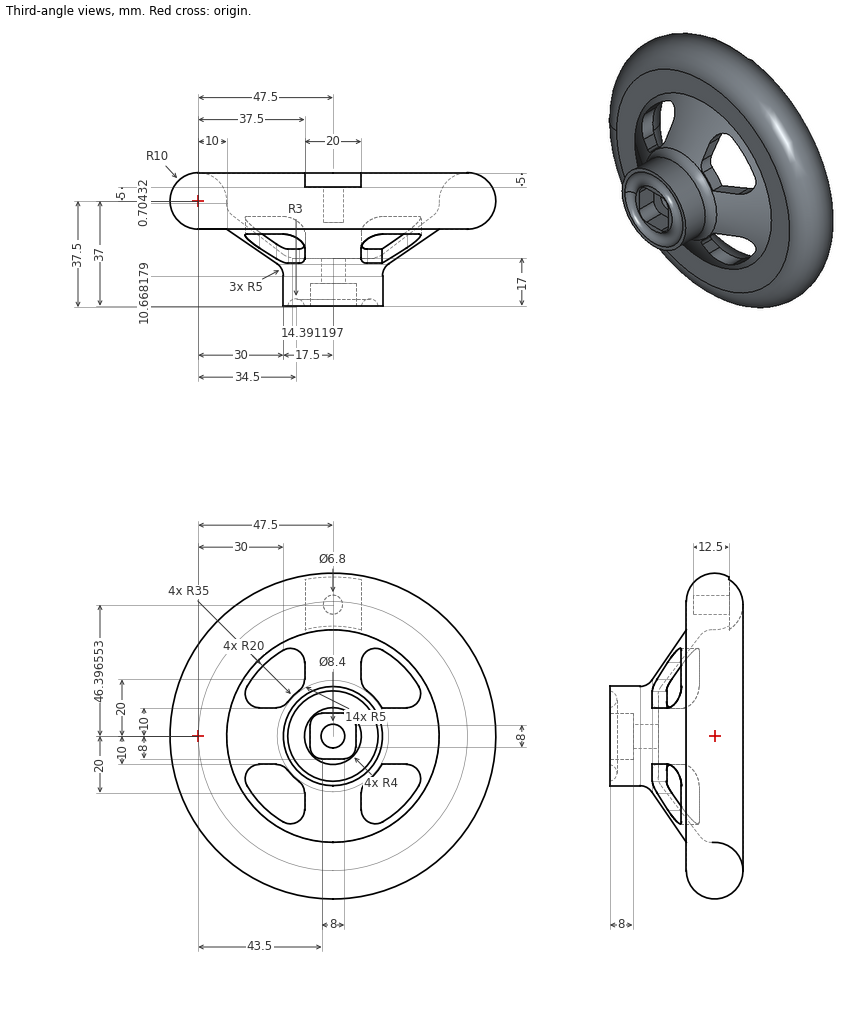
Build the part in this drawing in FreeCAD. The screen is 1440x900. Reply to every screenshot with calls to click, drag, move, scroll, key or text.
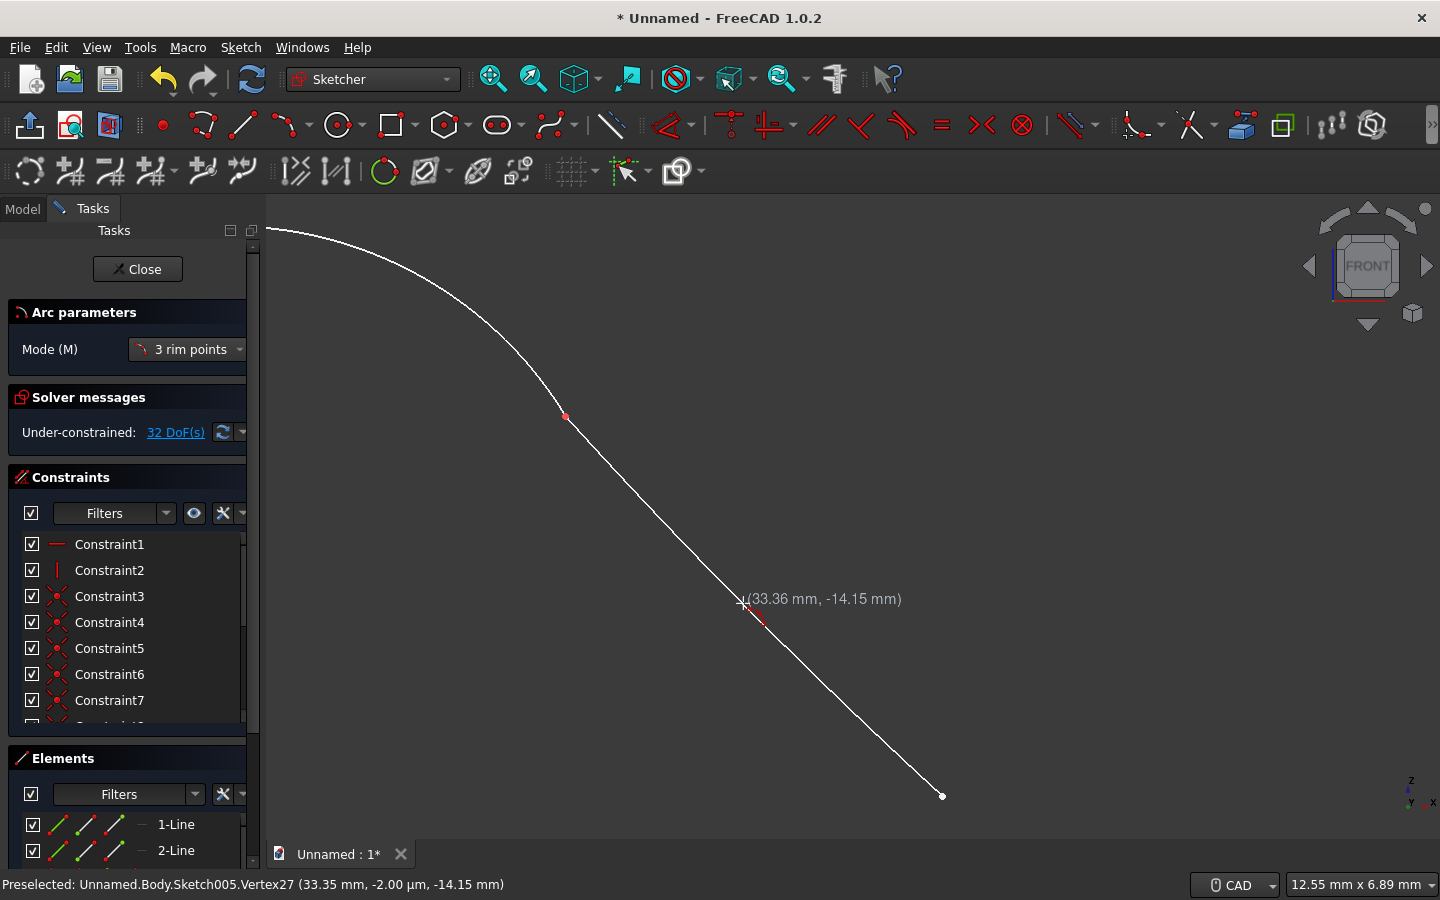
scroll(746, 616, down, 13)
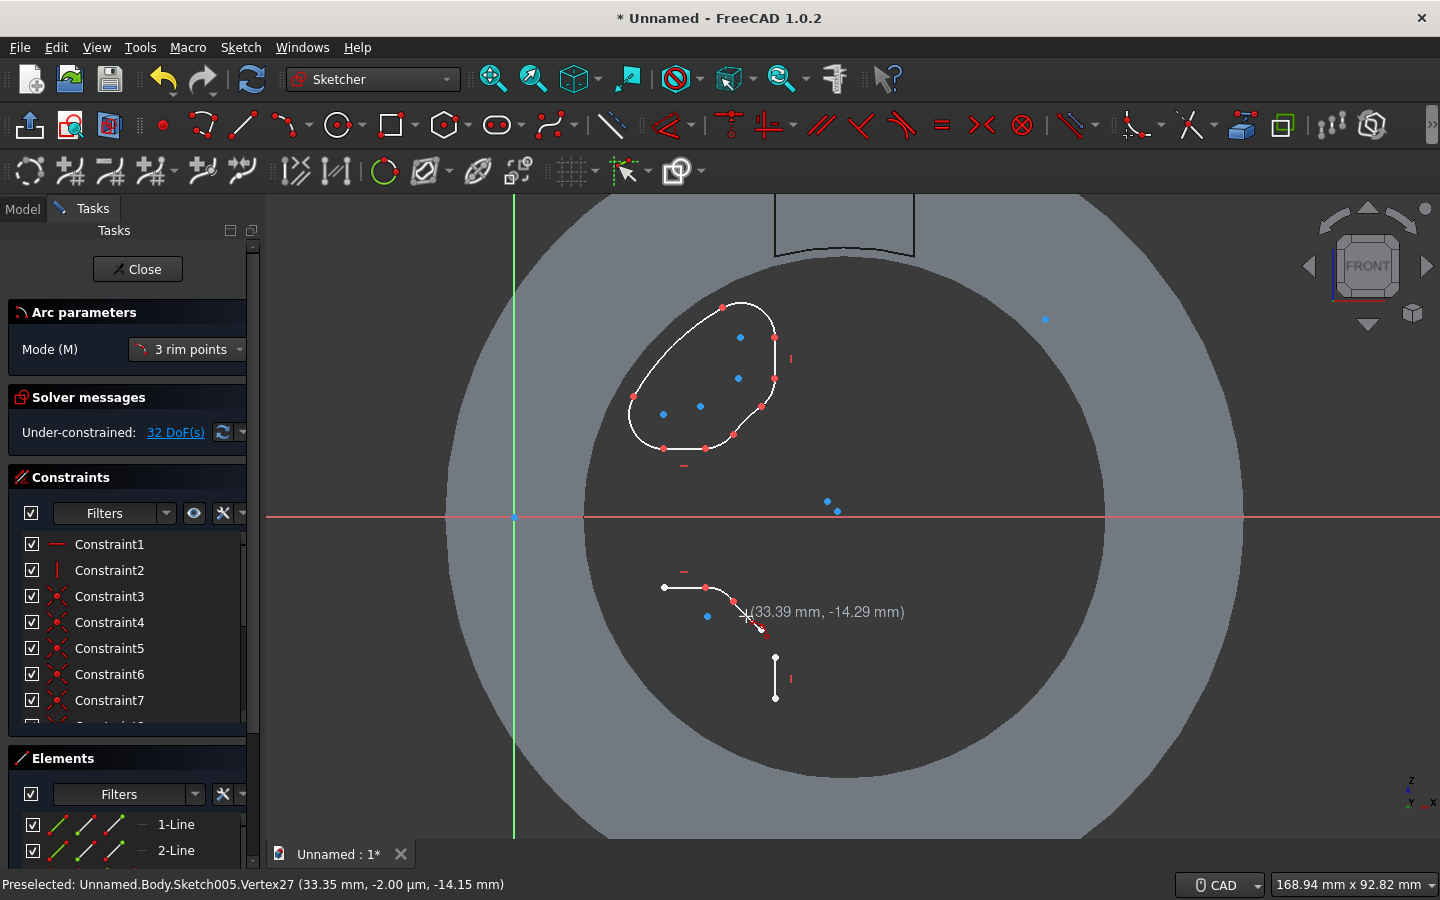
click(761, 630)
click(775, 658)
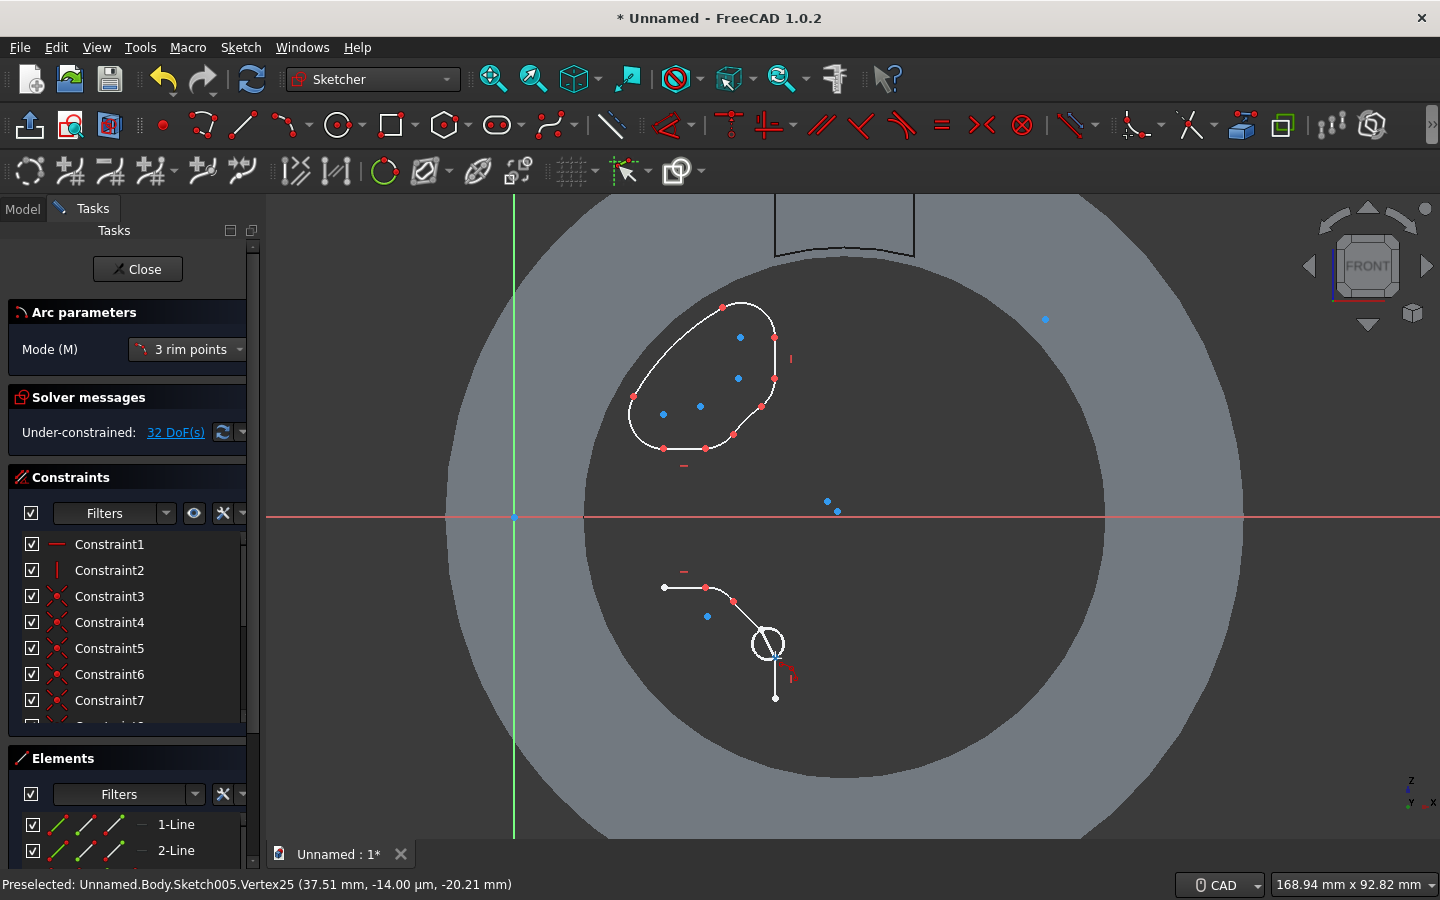
scroll(771, 641, up, 8)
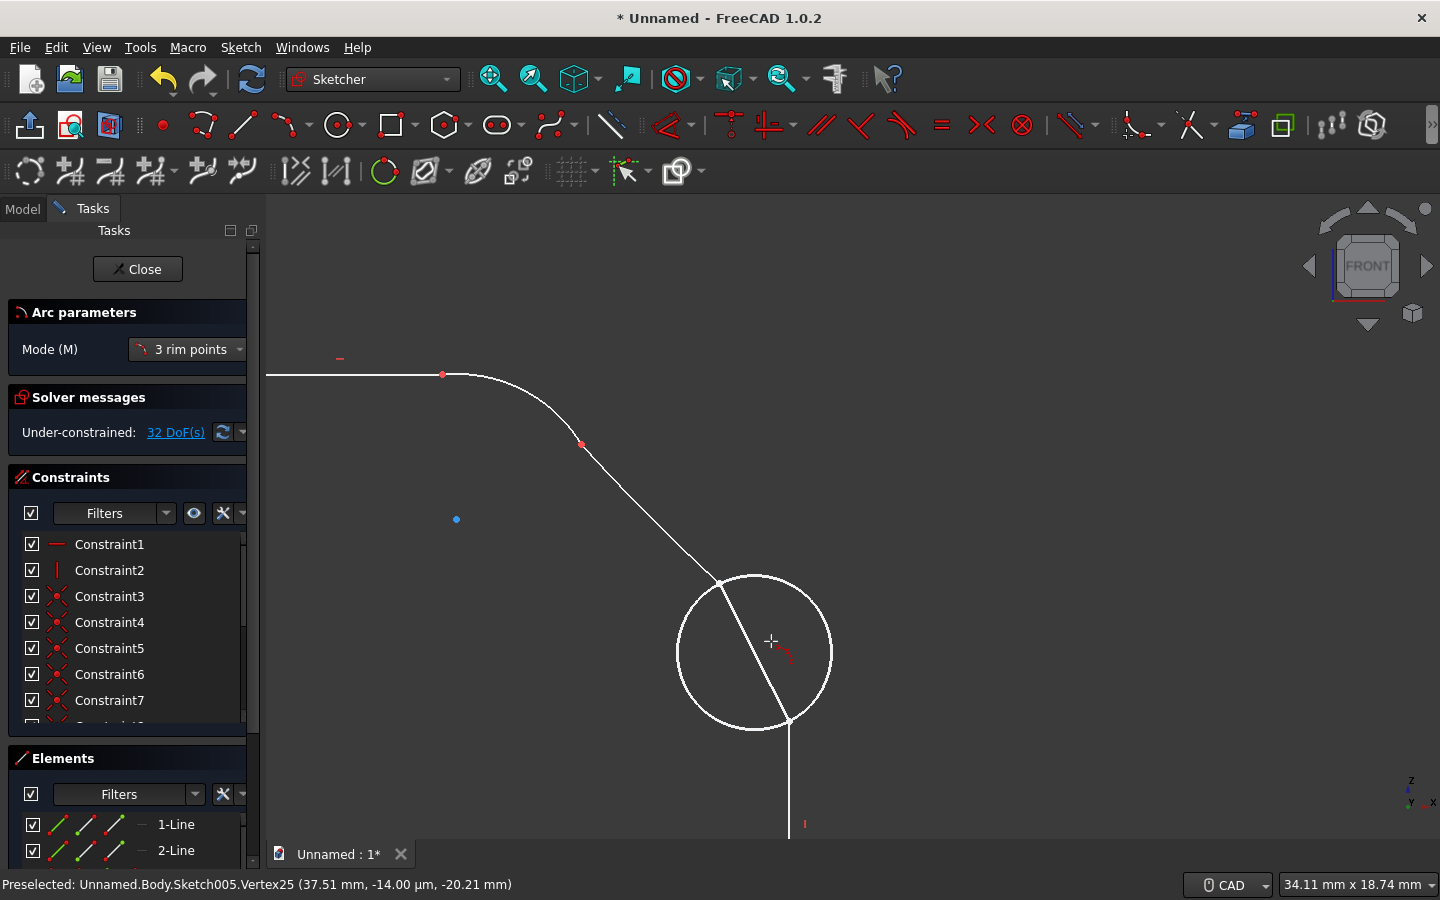
click(771, 637)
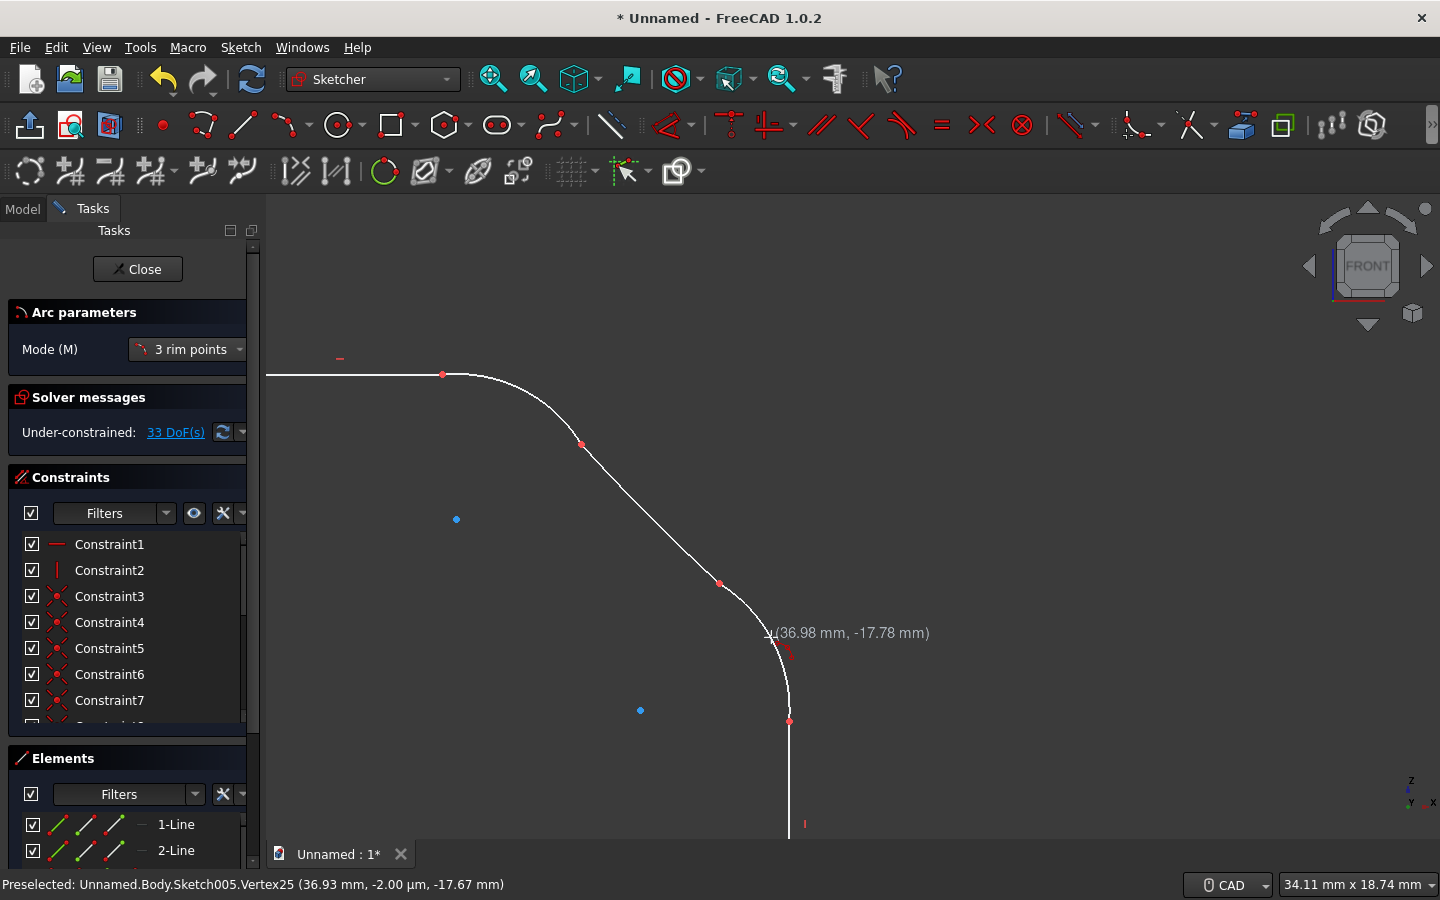
scroll(771, 641, down, 8)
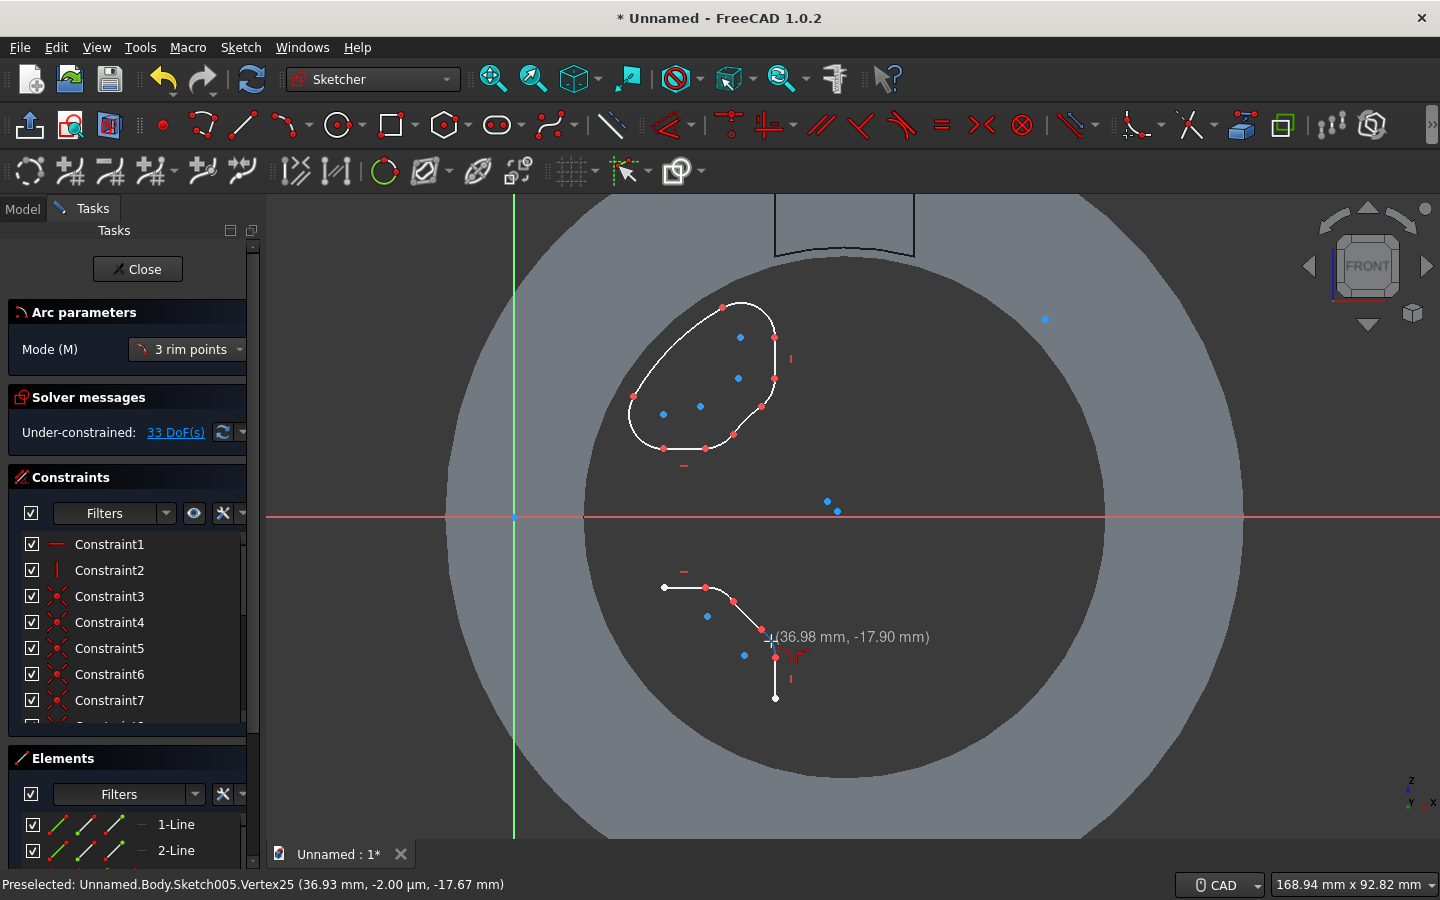
click(775, 699)
click(723, 728)
click(758, 728)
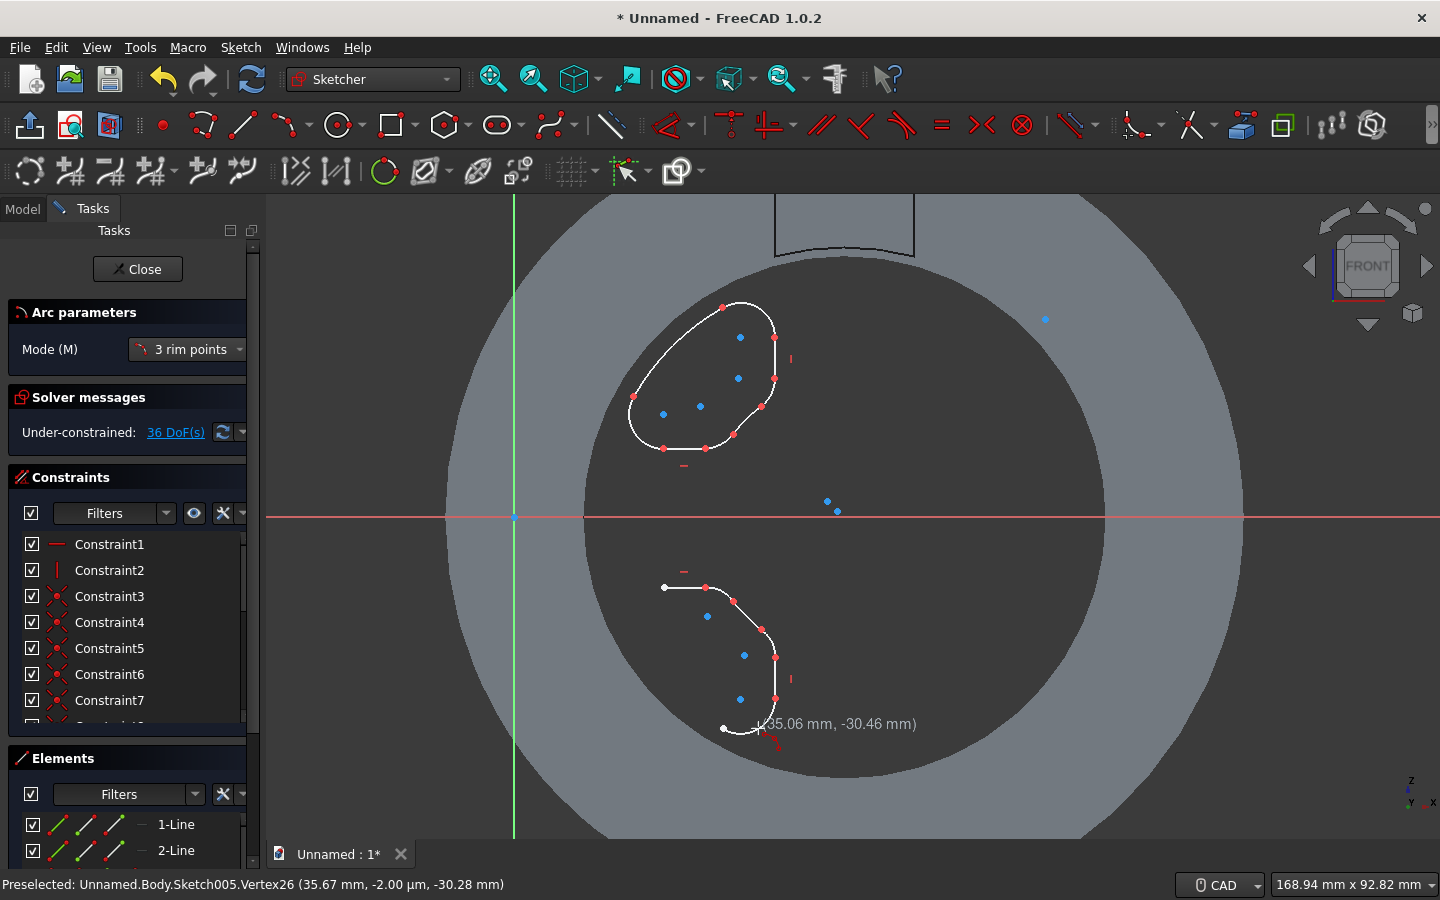
click(723, 729)
click(634, 639)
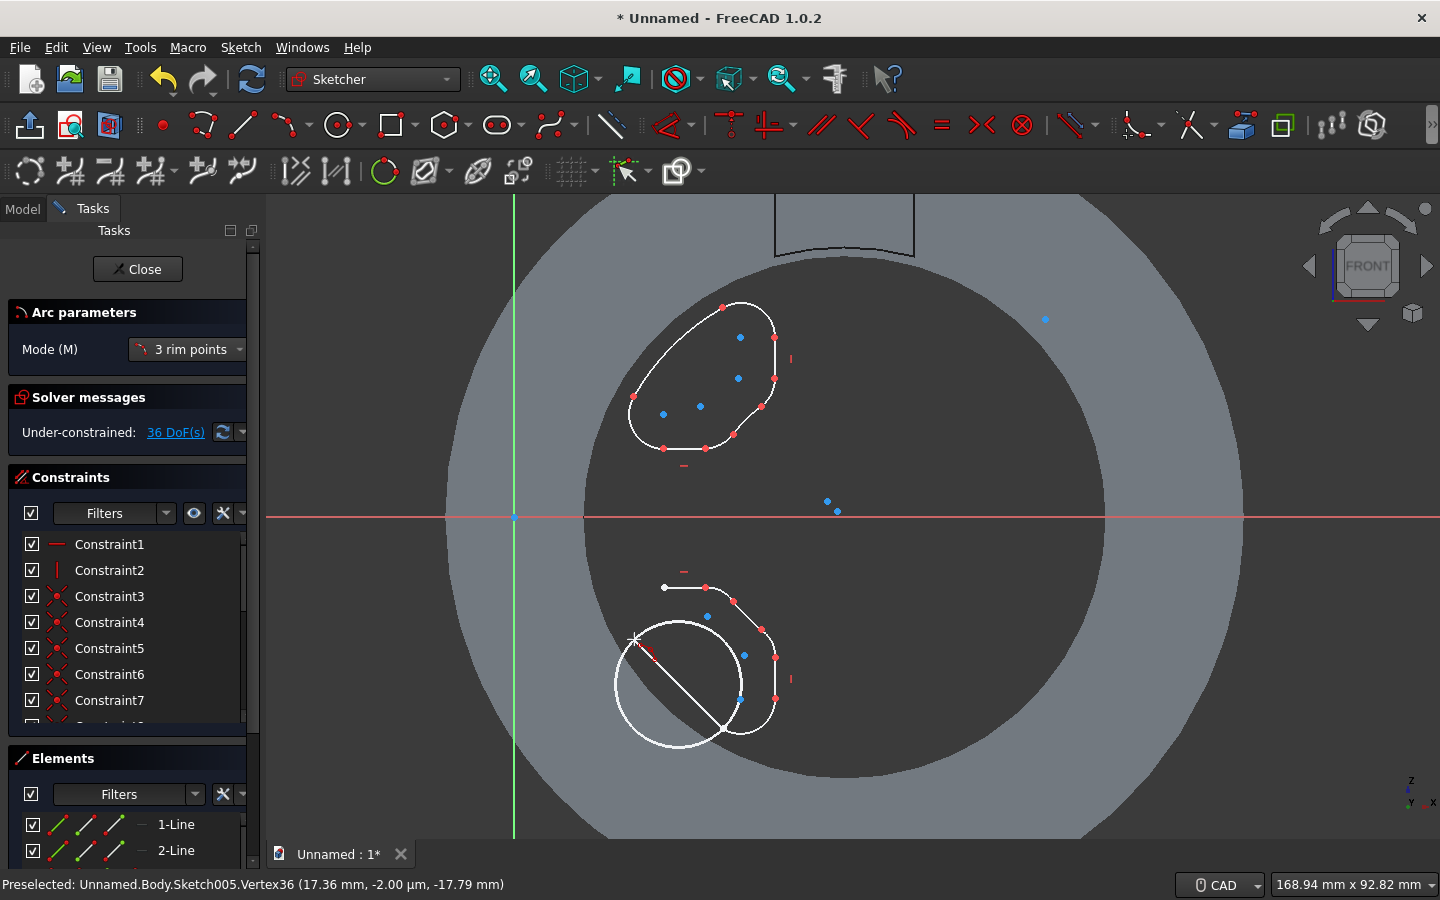
scroll(672, 689, up, 4)